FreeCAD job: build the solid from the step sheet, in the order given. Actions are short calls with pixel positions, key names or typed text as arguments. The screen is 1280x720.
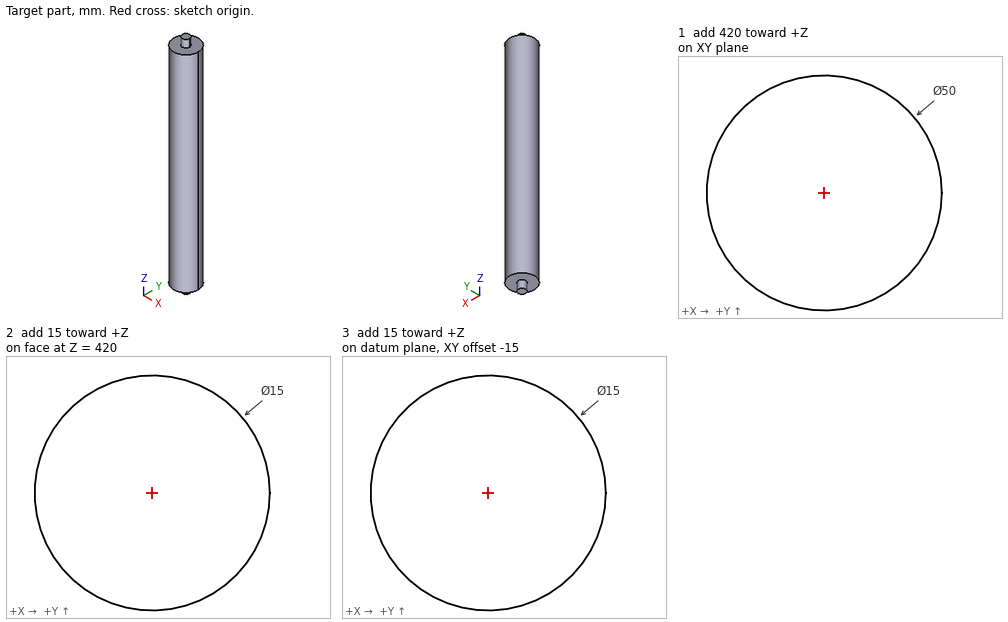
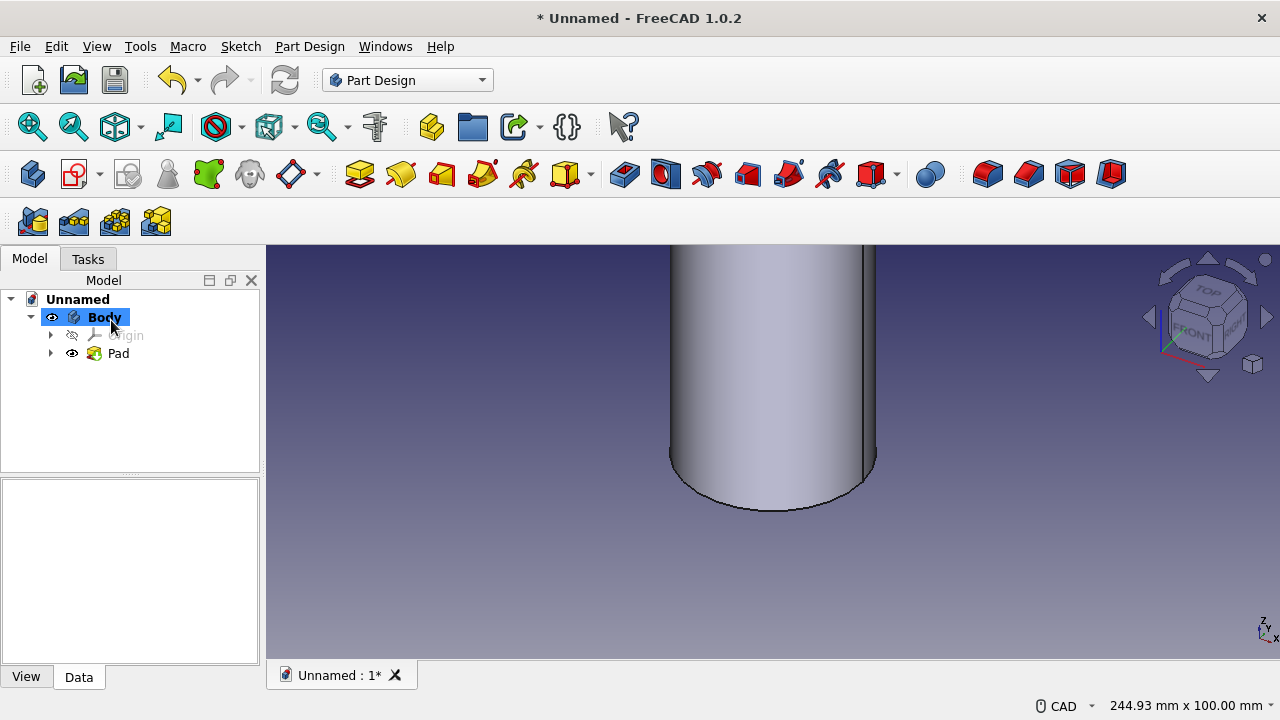
key(v)
key(f)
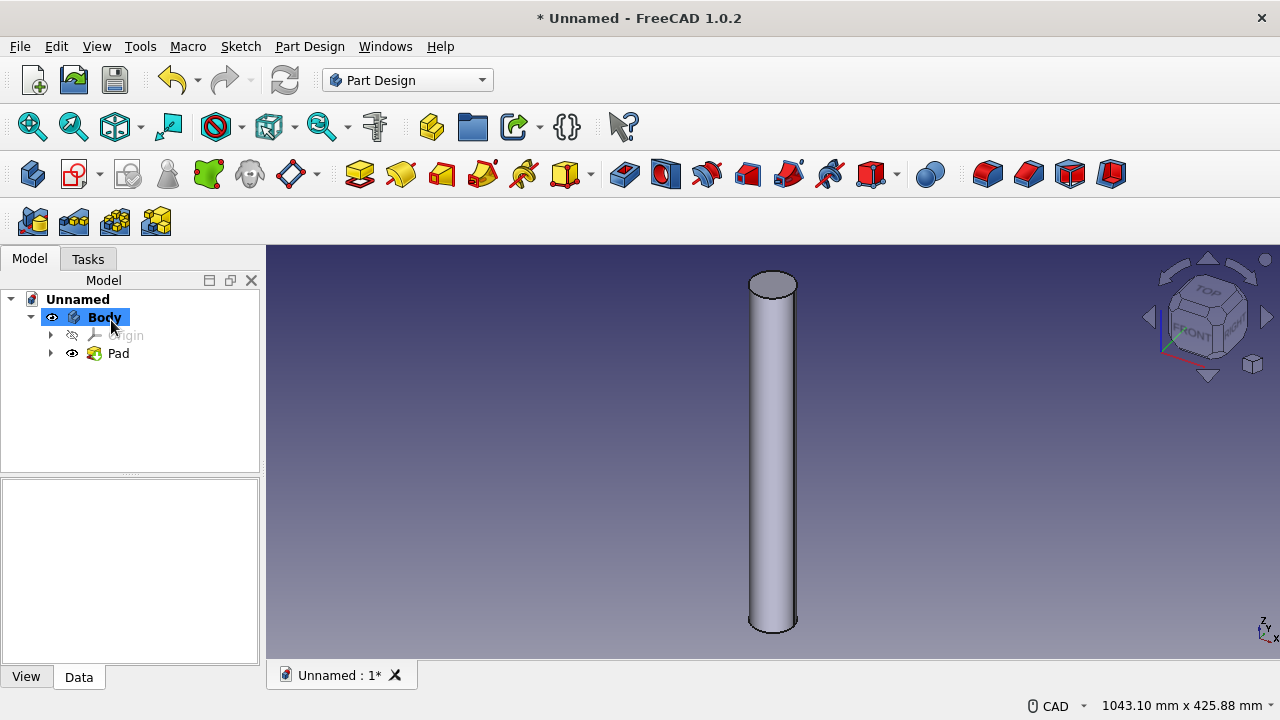
click(773, 284)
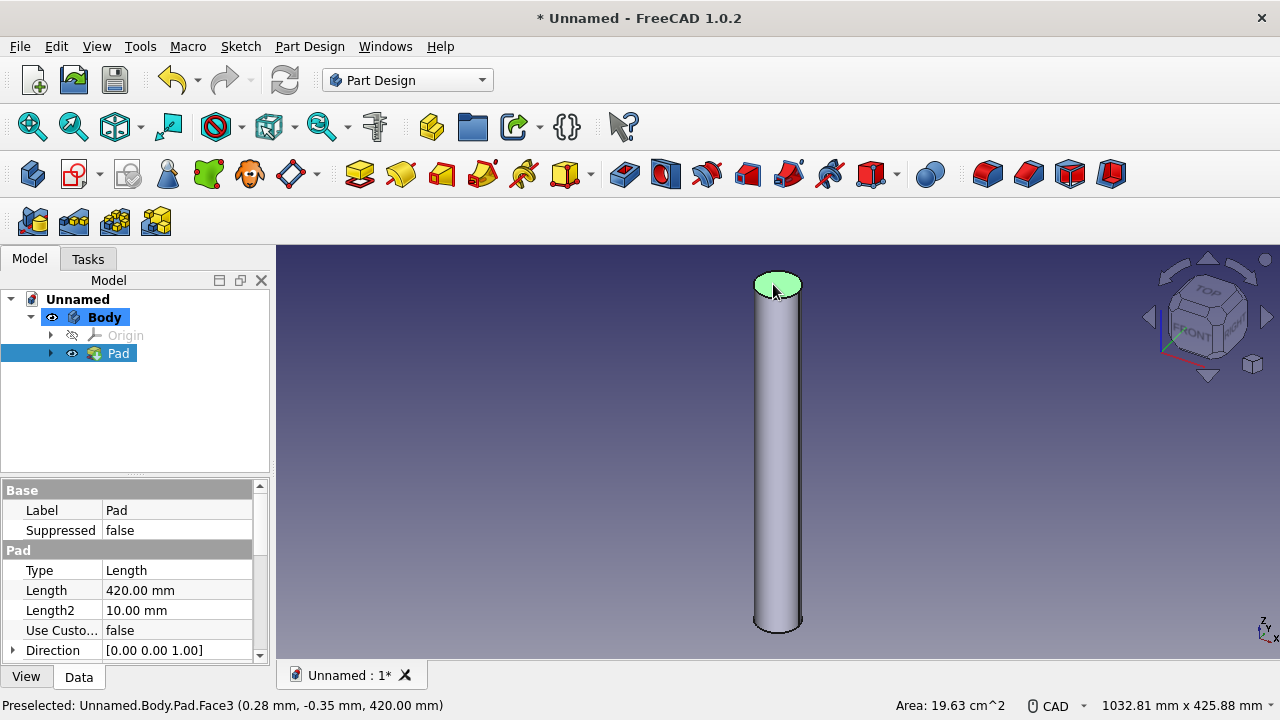
click(74, 174)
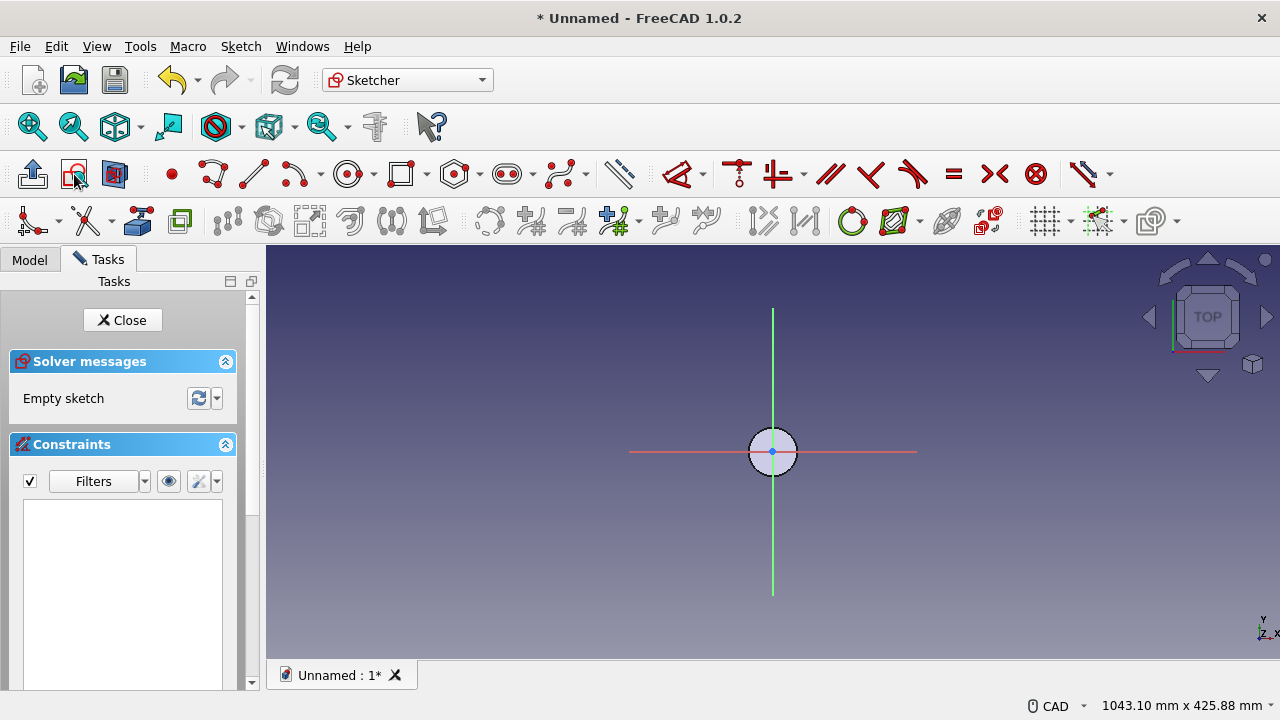
scroll(777, 452, up, 14)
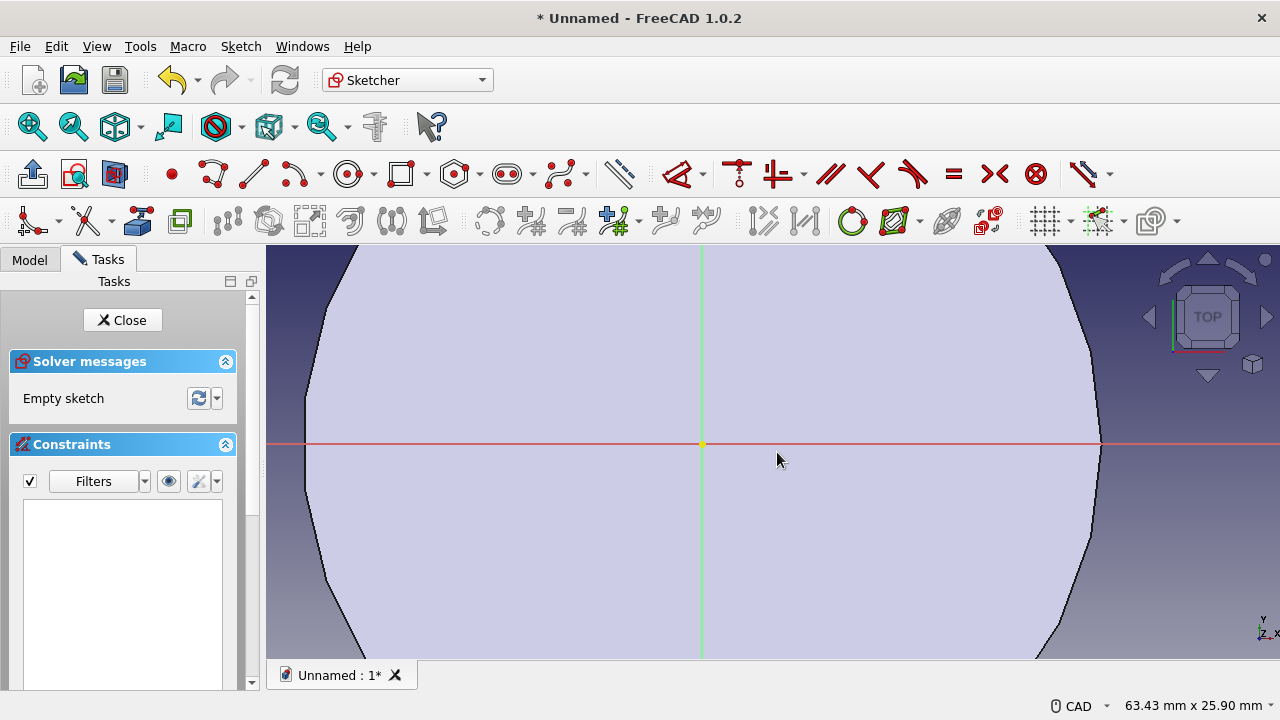
key(g)
key(c)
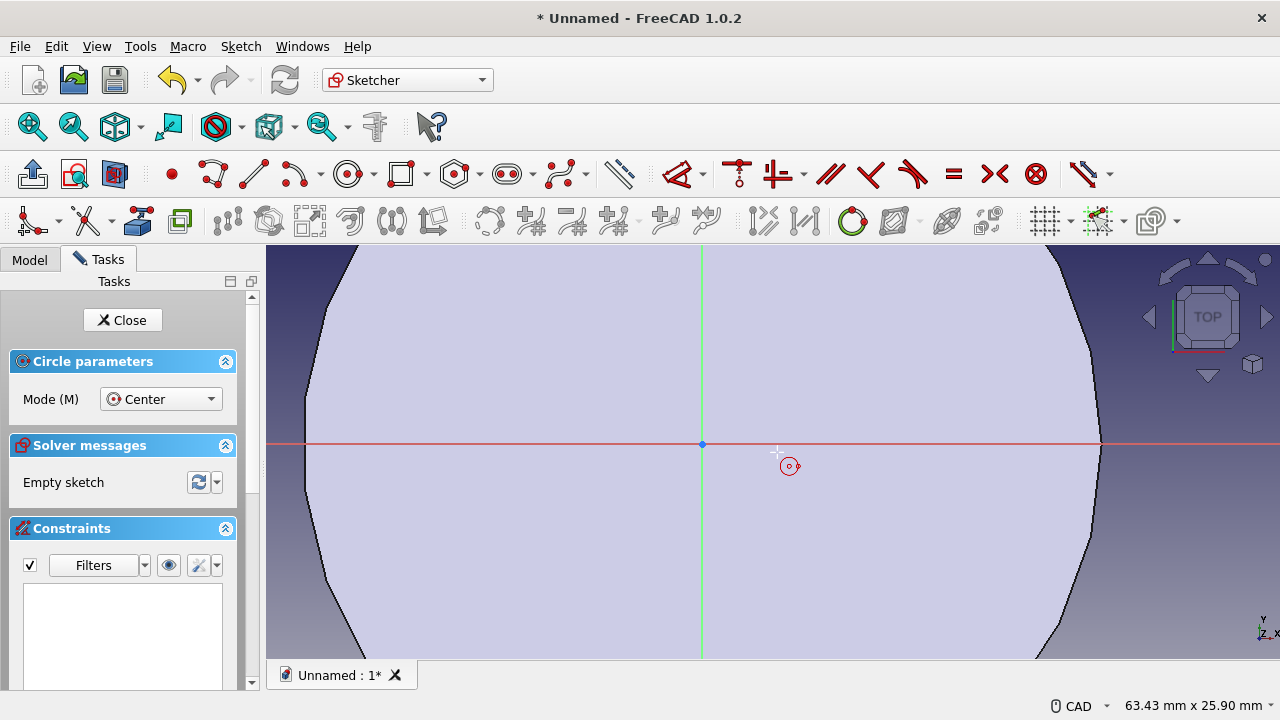
click(702, 444)
move(787, 359)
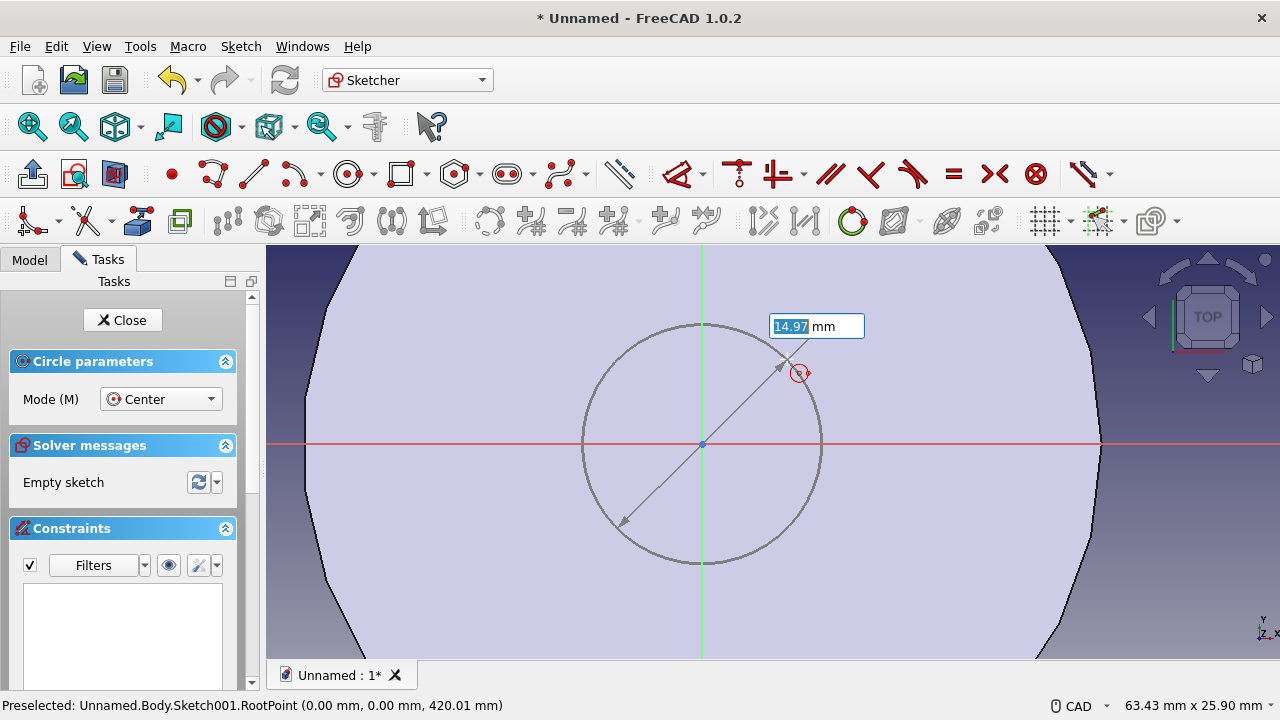
text(15)
key(Return)
key(Escape)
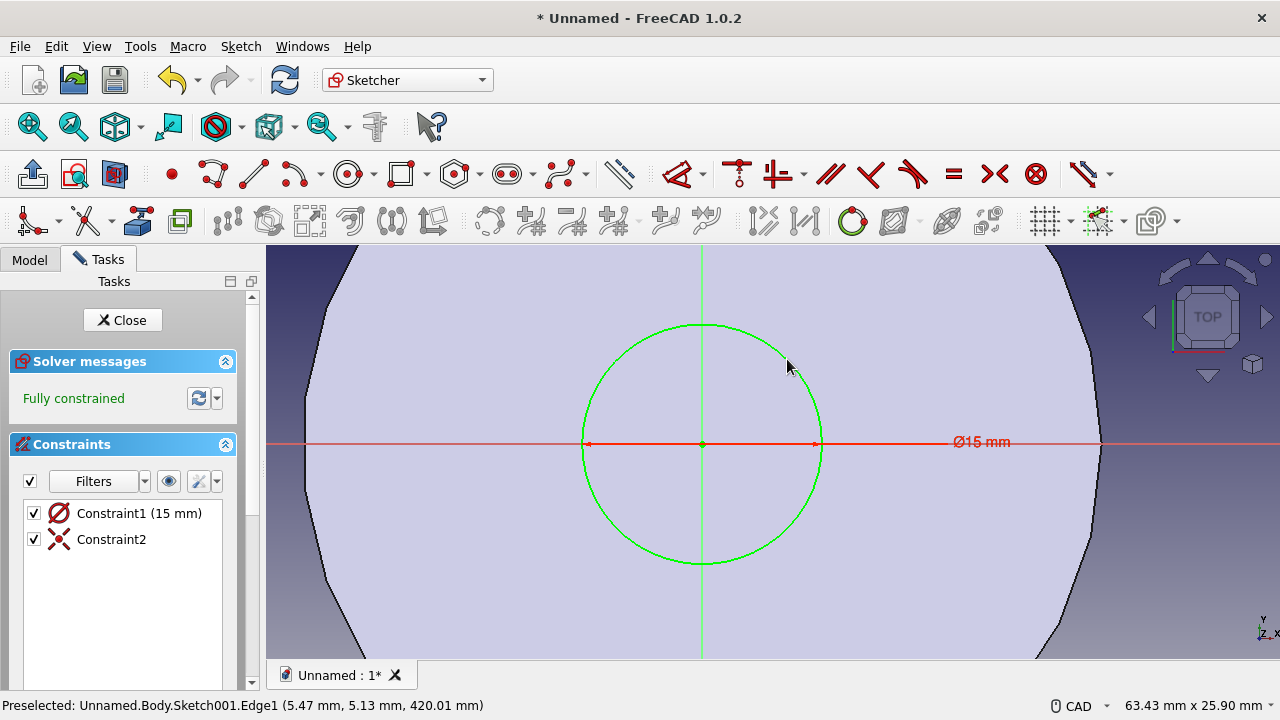
click(123, 320)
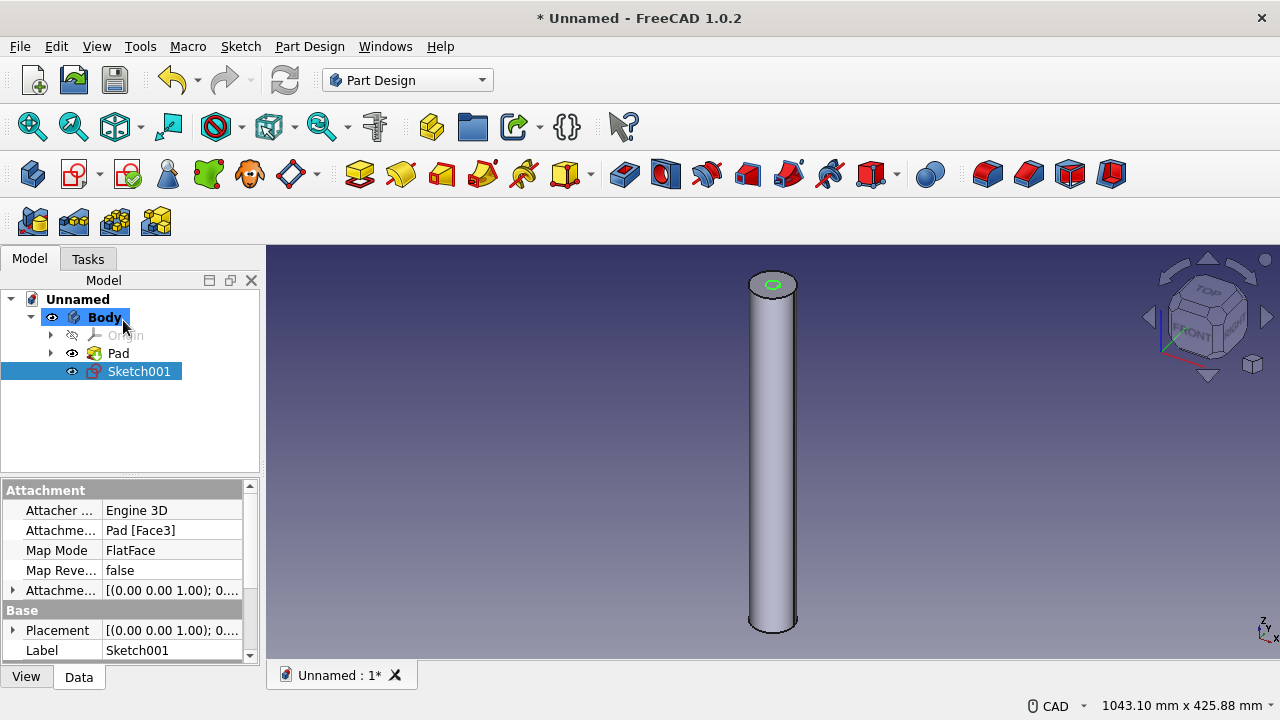
click(360, 174)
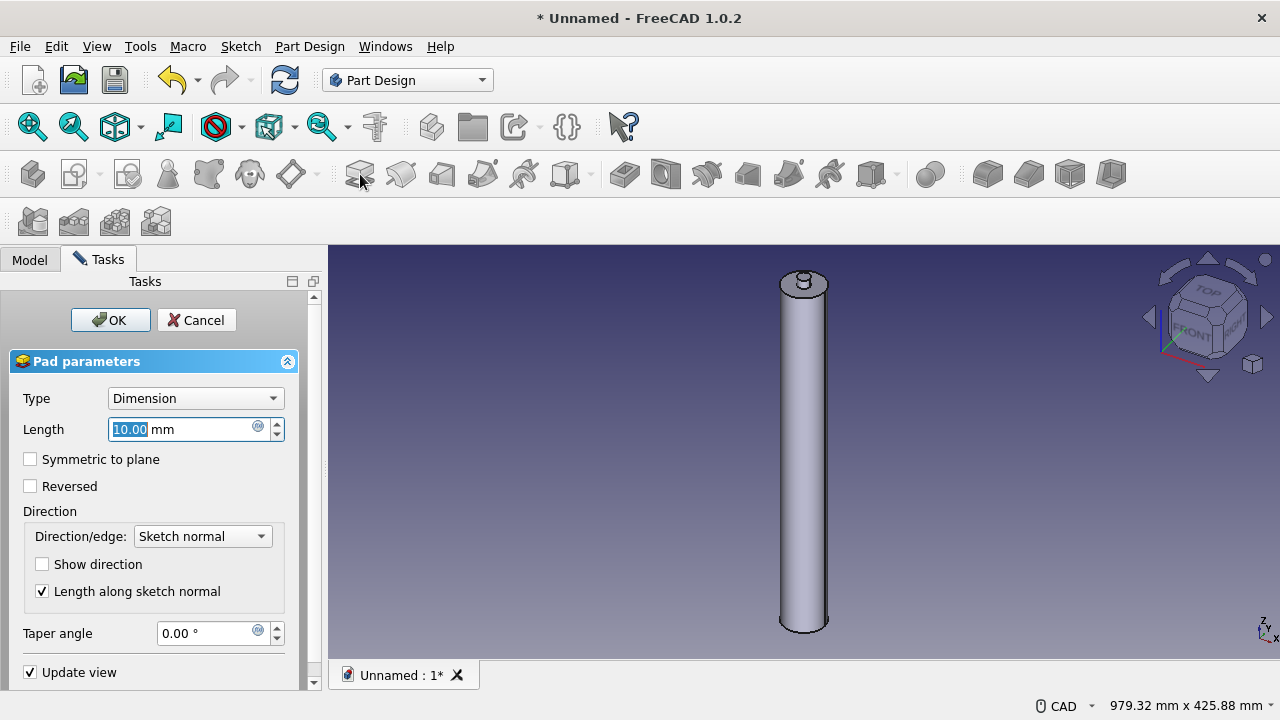
text(15)
key(Tab)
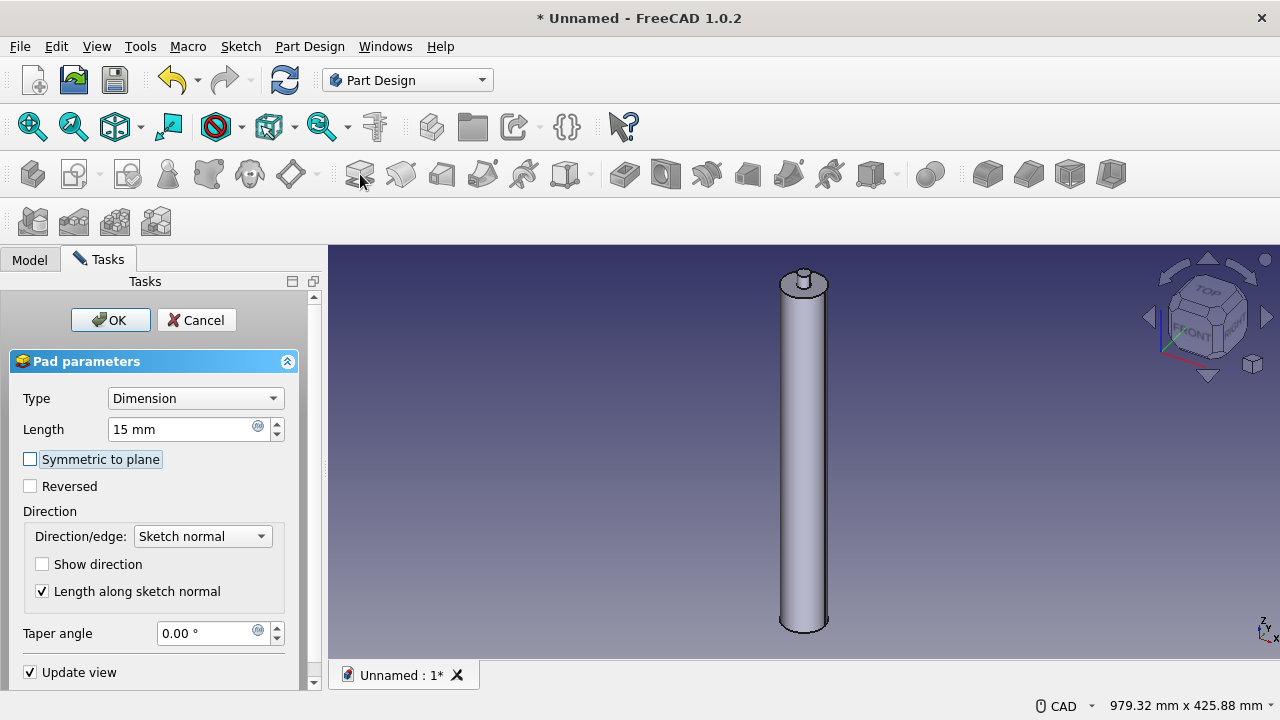
click(111, 320)